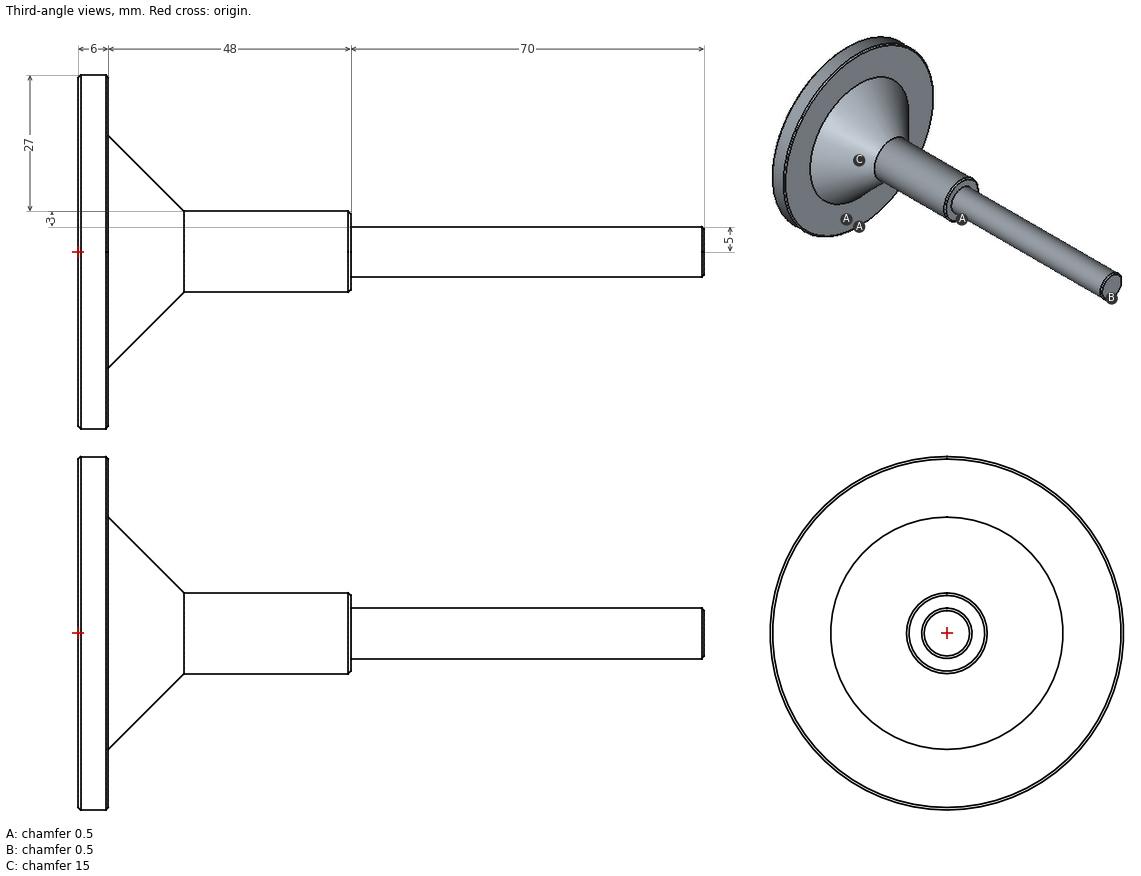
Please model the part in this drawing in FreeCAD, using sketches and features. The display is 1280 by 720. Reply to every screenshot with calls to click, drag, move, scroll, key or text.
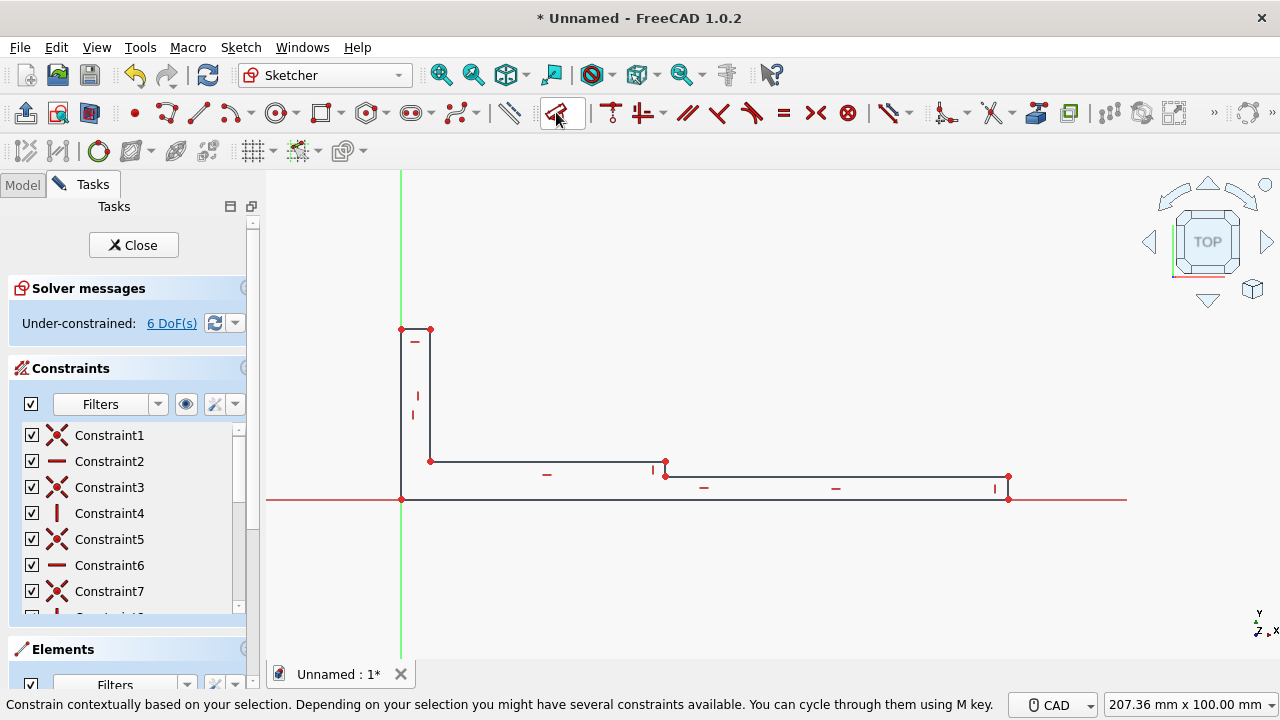
scroll(1008, 491, up, 3)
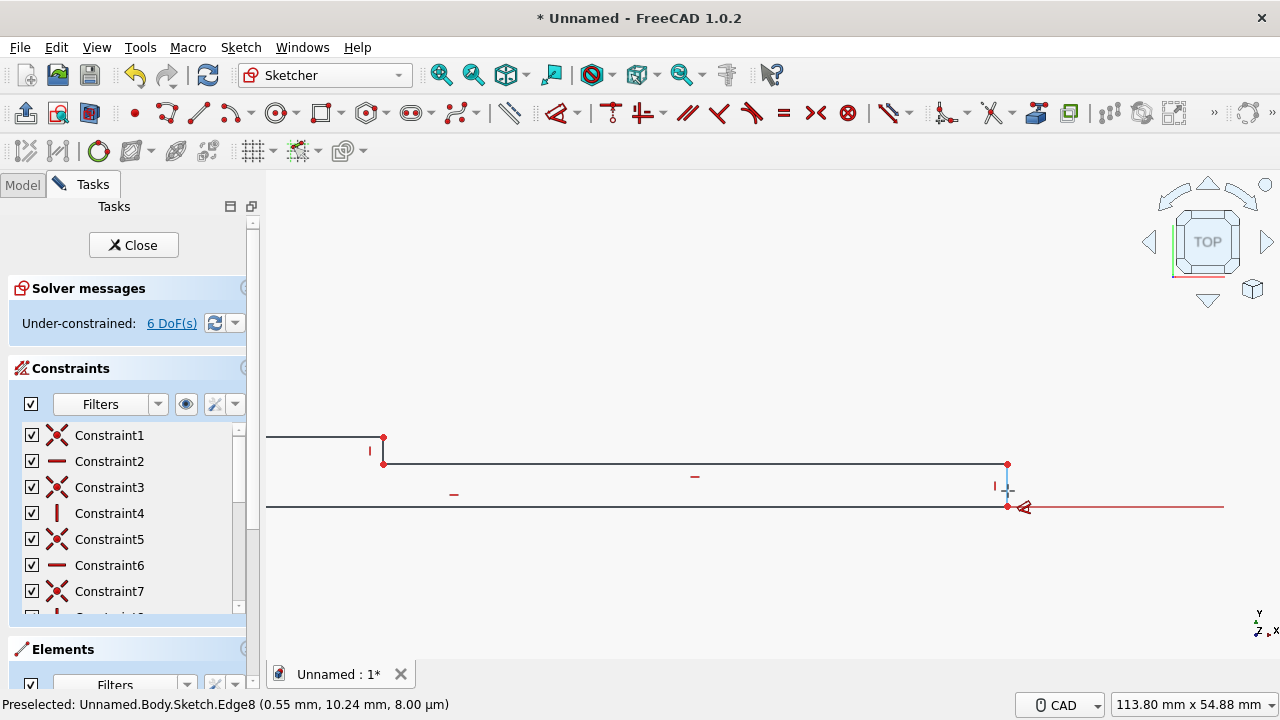
click(1007, 490)
click(1041, 486)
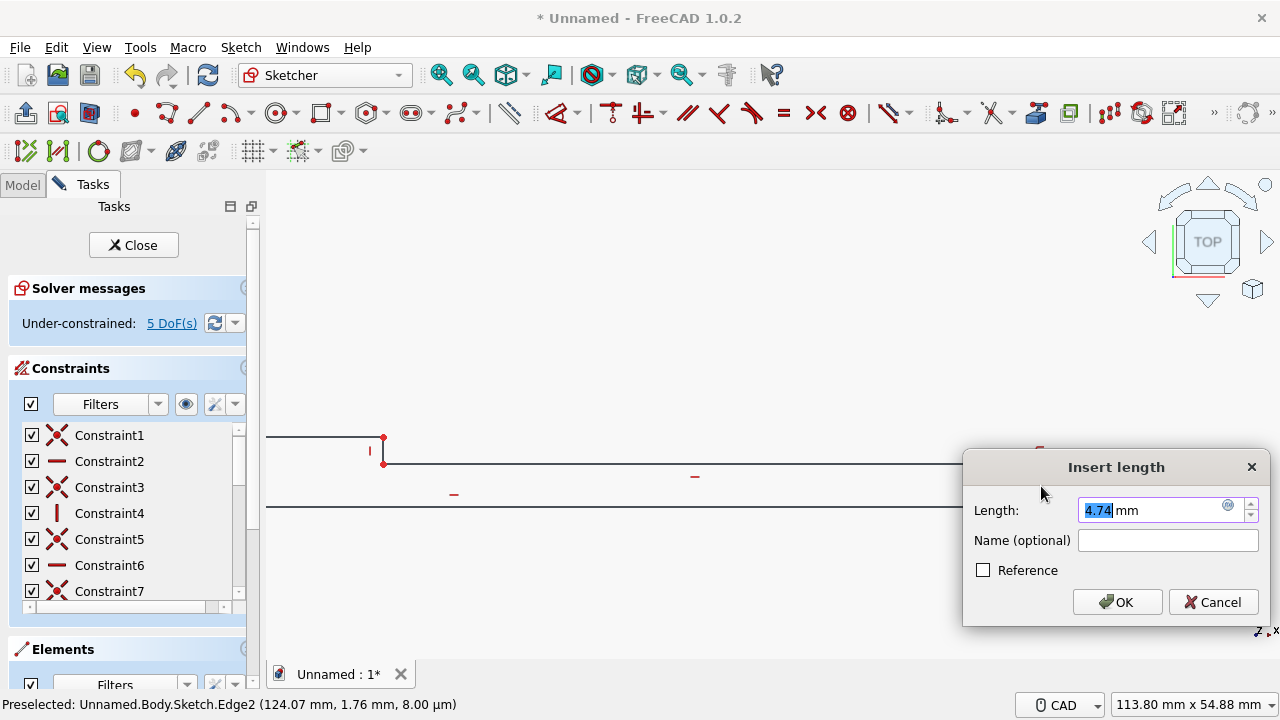
text(5)
key(Return)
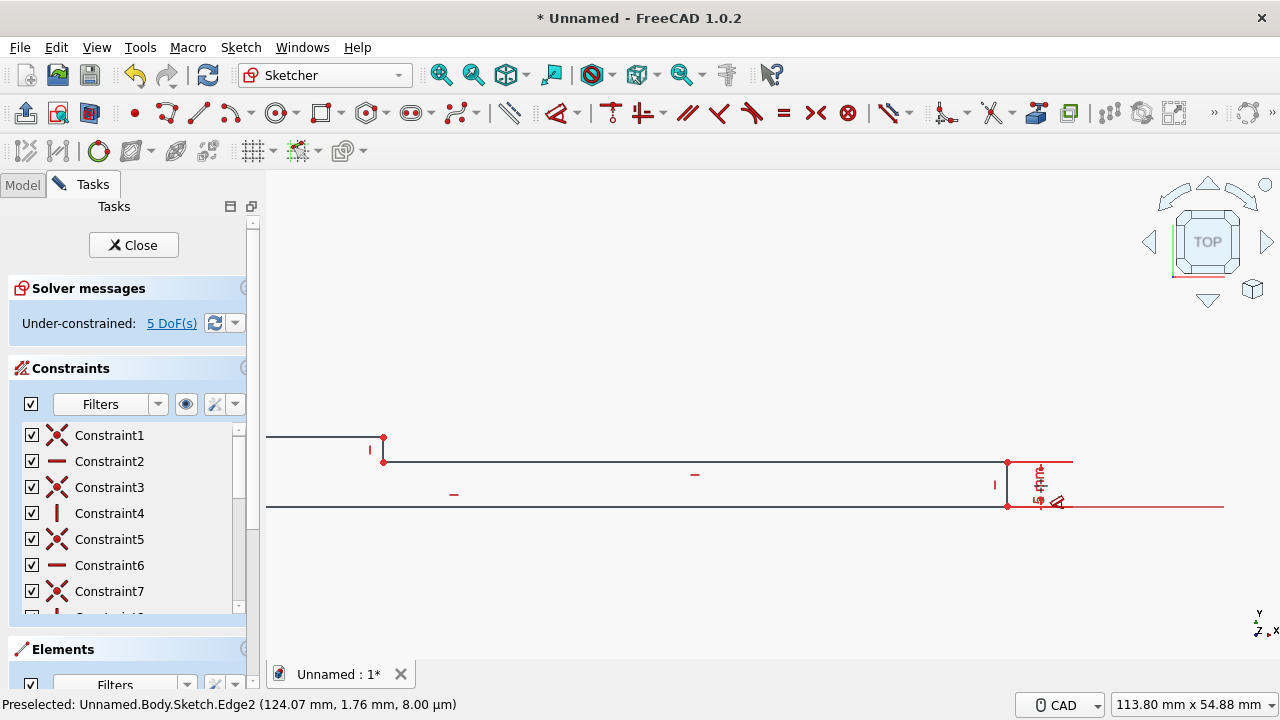
scroll(383, 452, up, 2)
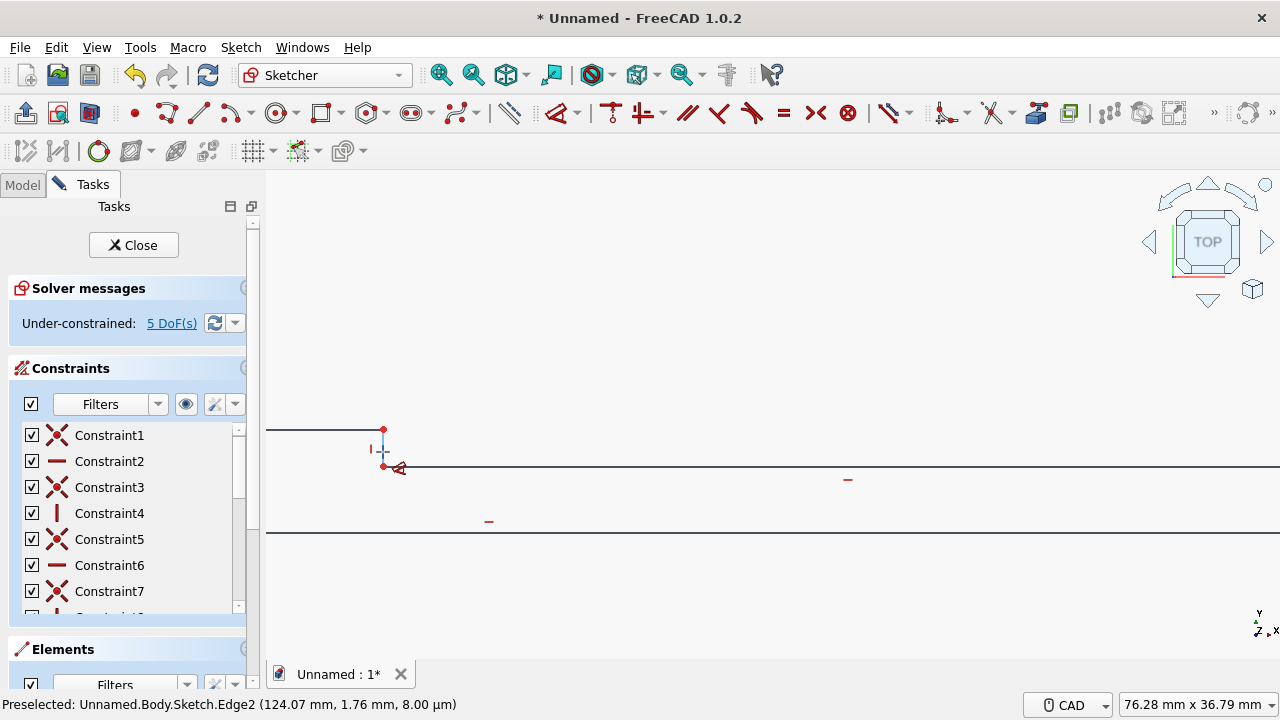
click(383, 452)
click(349, 448)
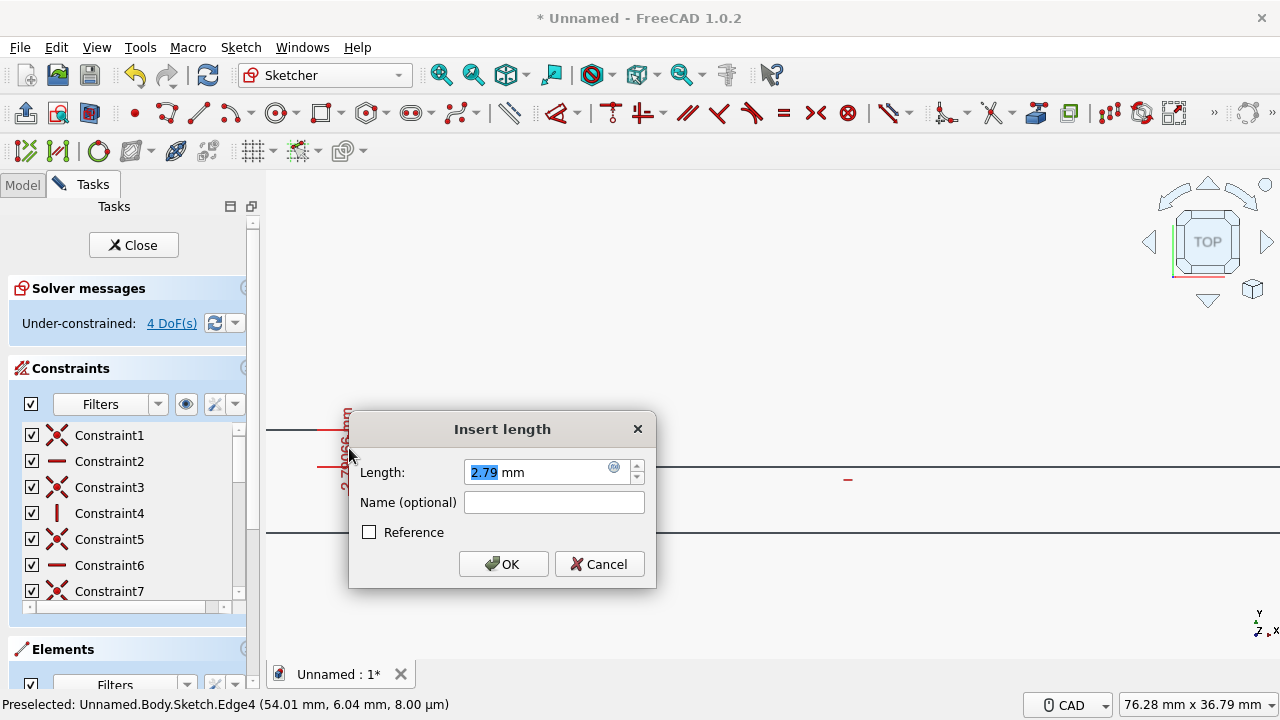
text(3)
key(Return)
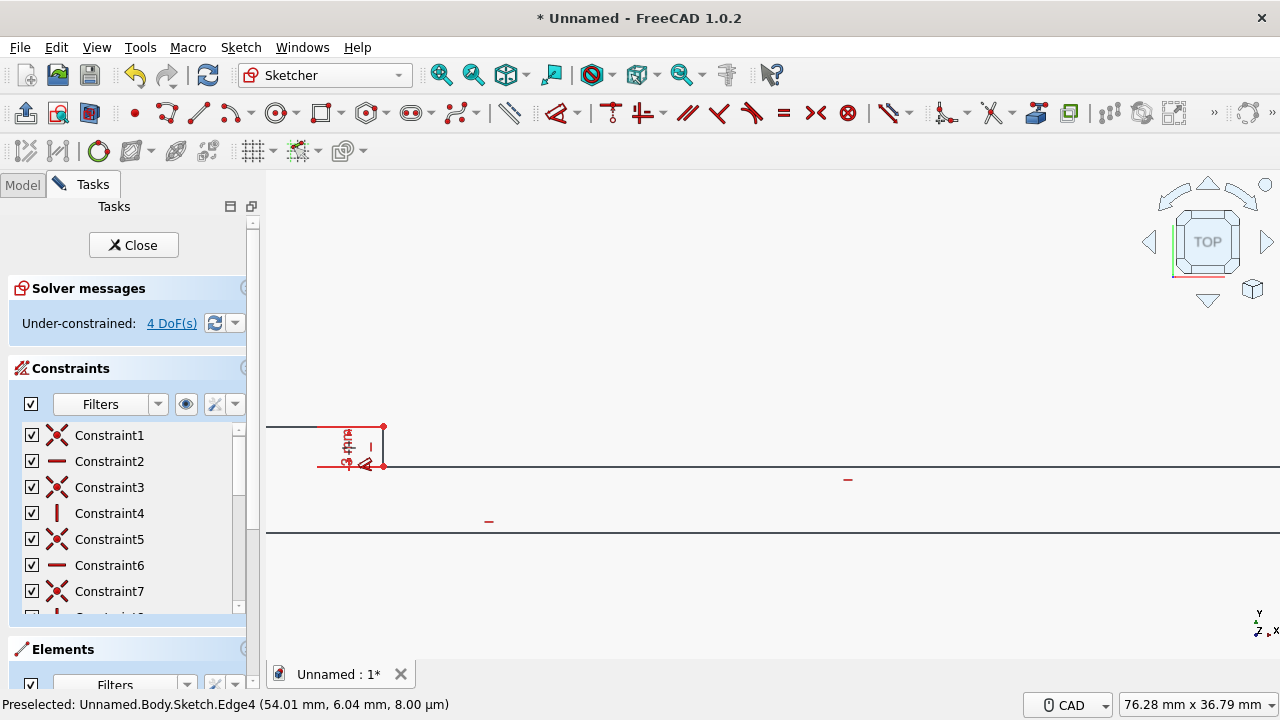
scroll(830, 481, down, 5)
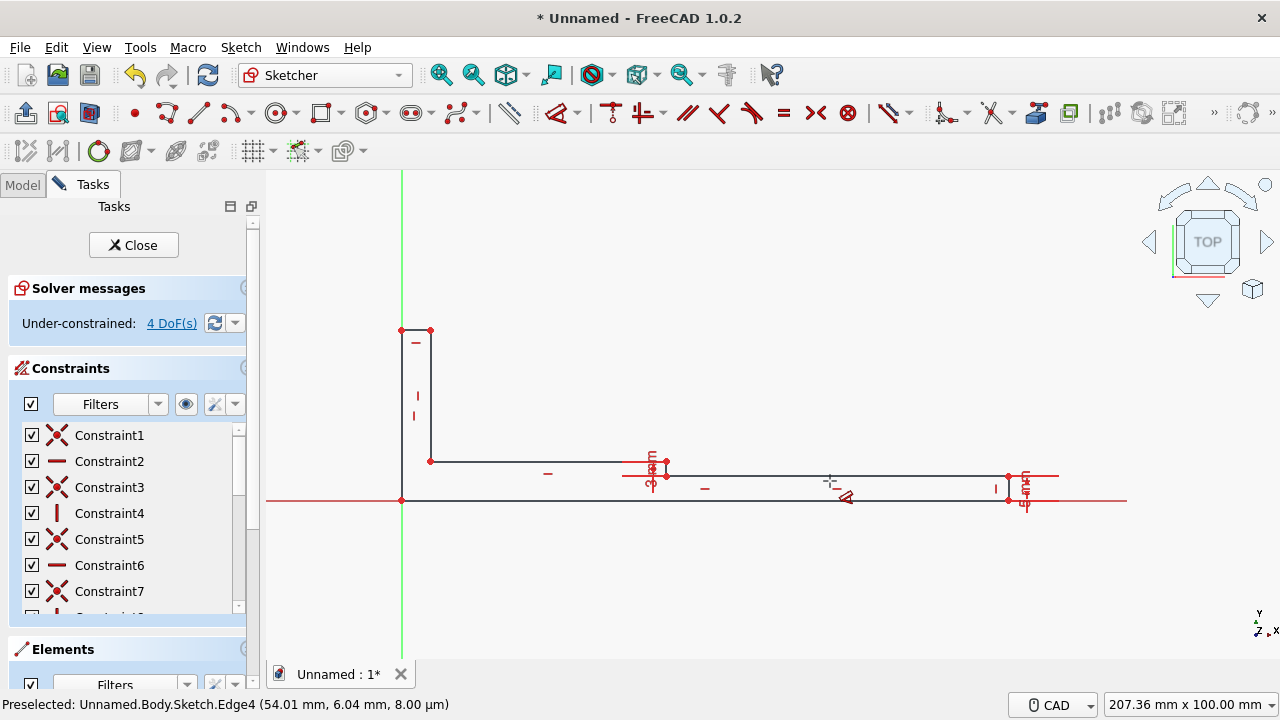
scroll(422, 330, up, 3)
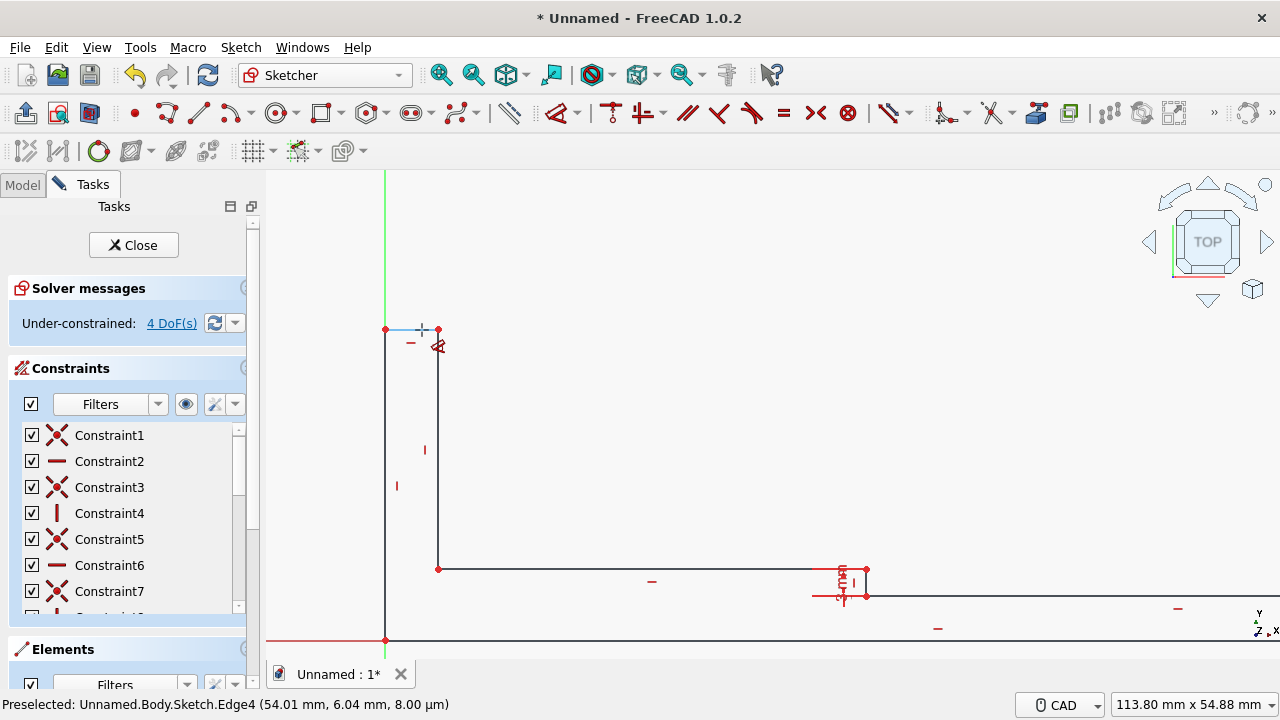
click(422, 330)
click(412, 296)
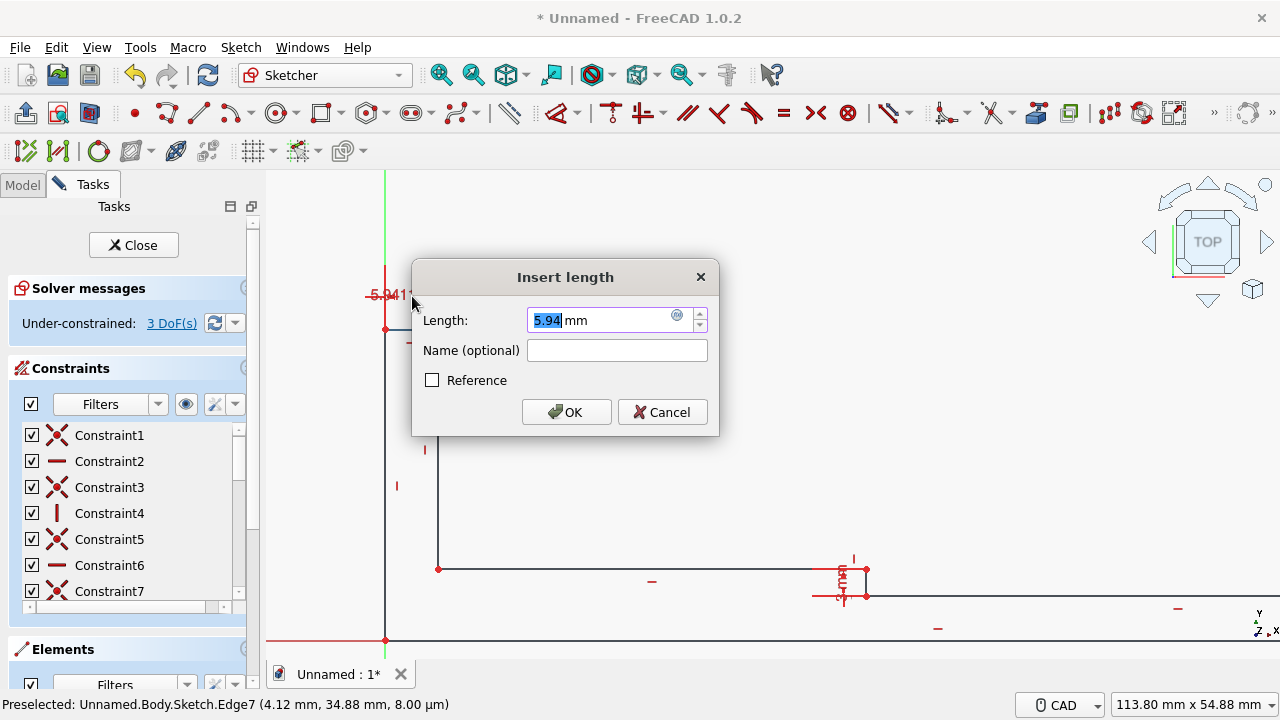
text(6)
key(Return)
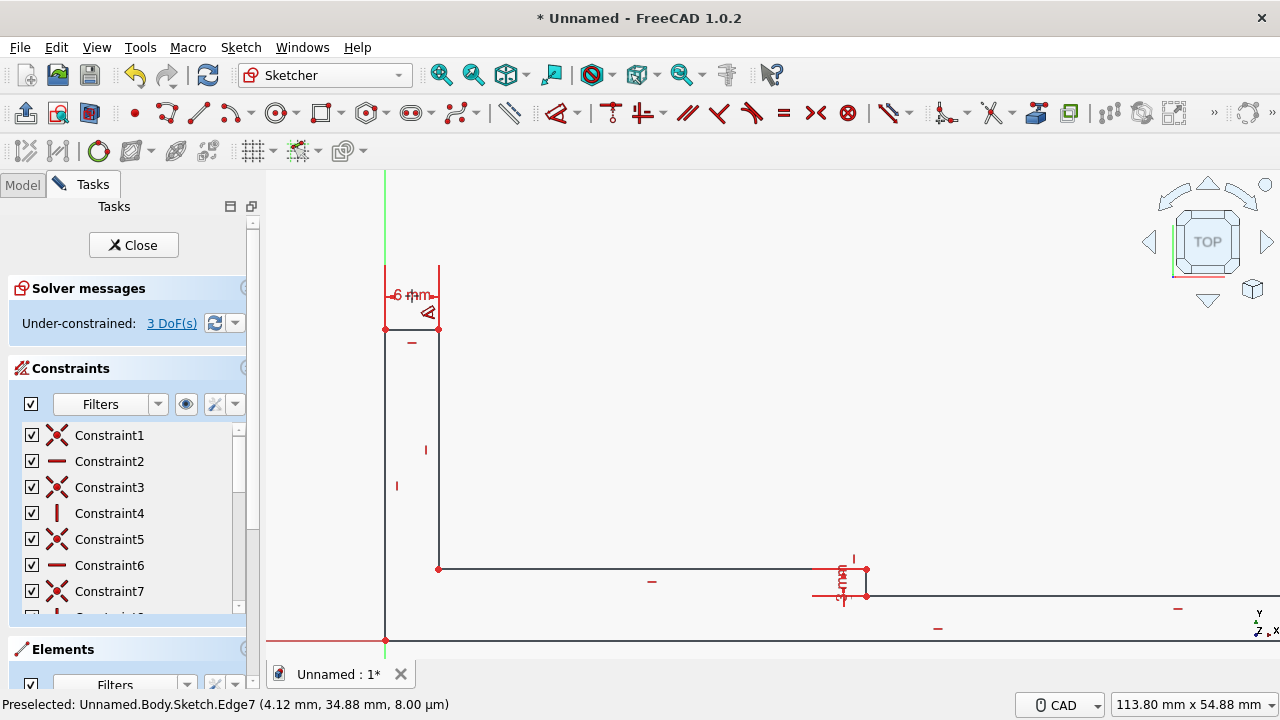
click(1054, 596)
click(991, 562)